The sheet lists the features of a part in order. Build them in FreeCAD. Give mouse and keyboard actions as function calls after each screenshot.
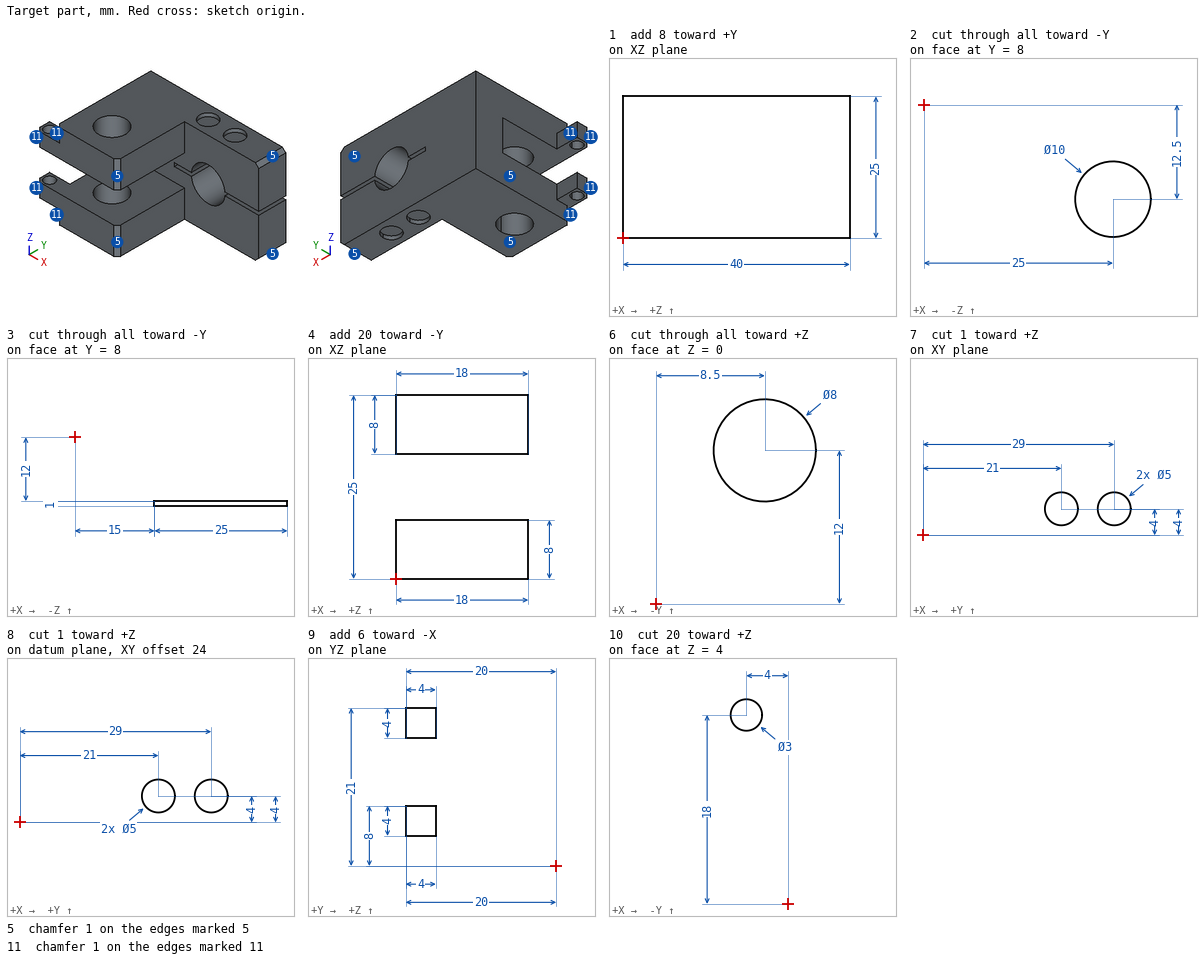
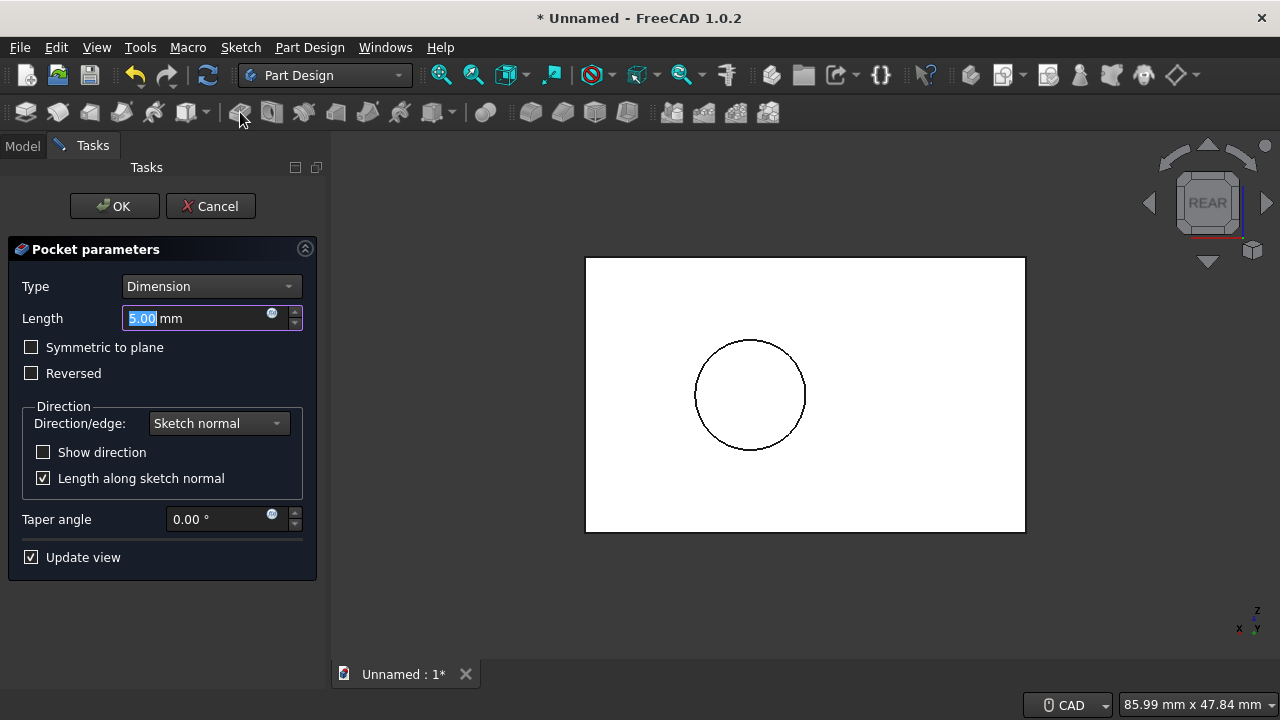
click(212, 286)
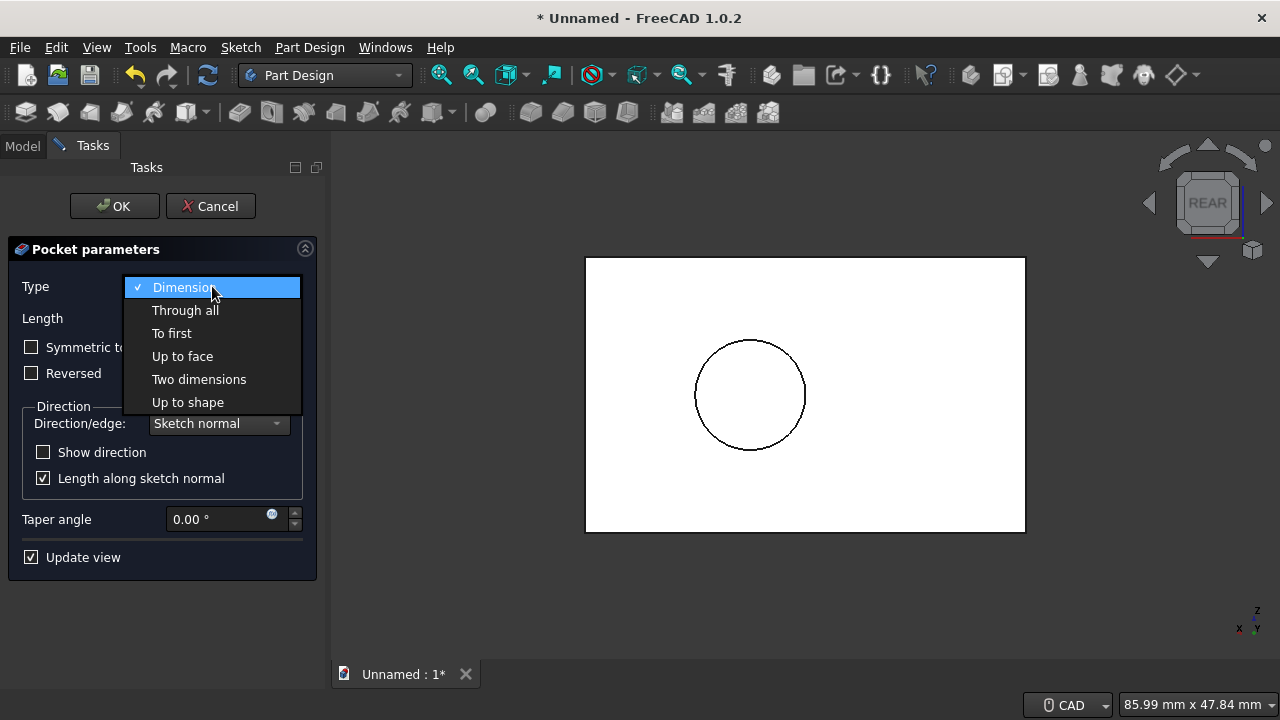
click(212, 310)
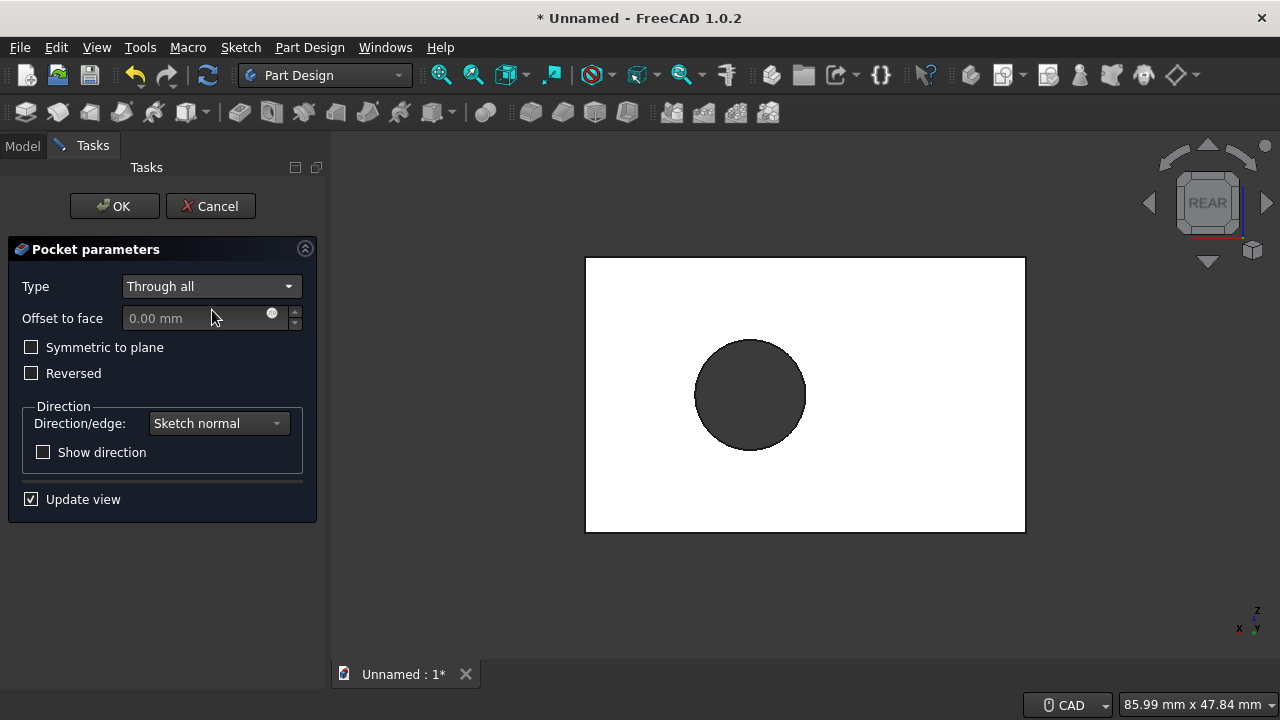
click(115, 206)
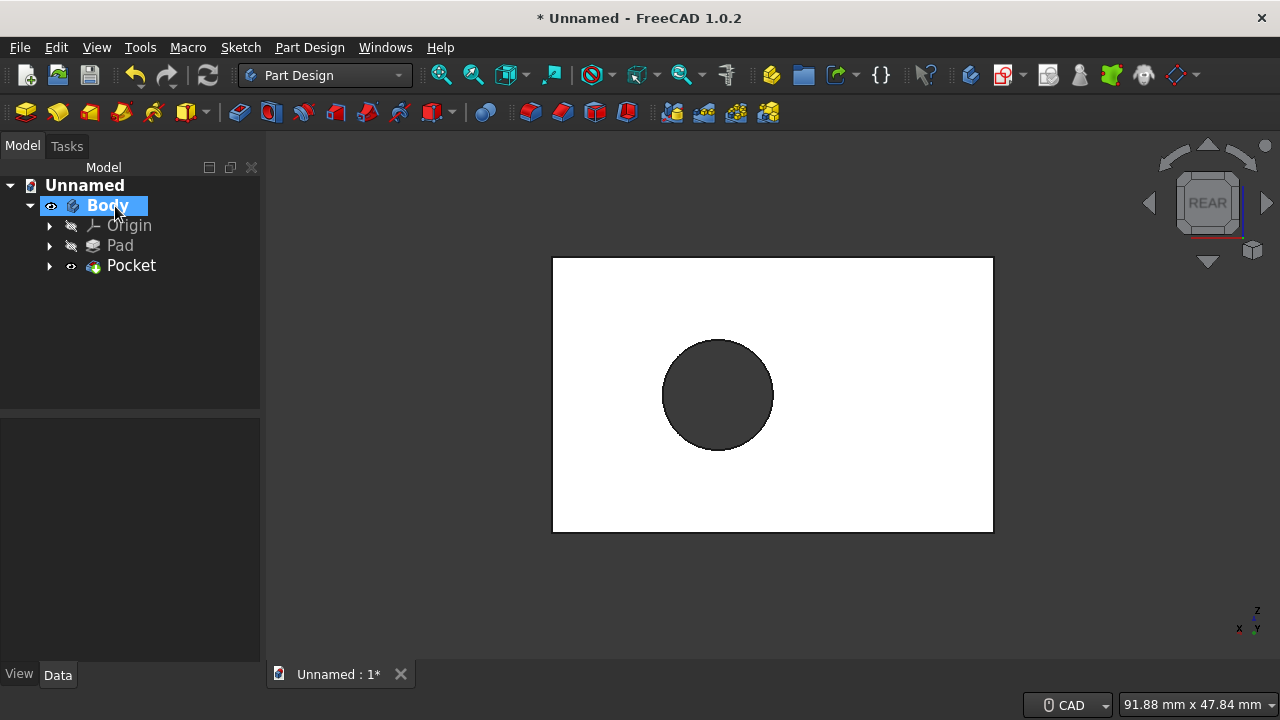
click(899, 355)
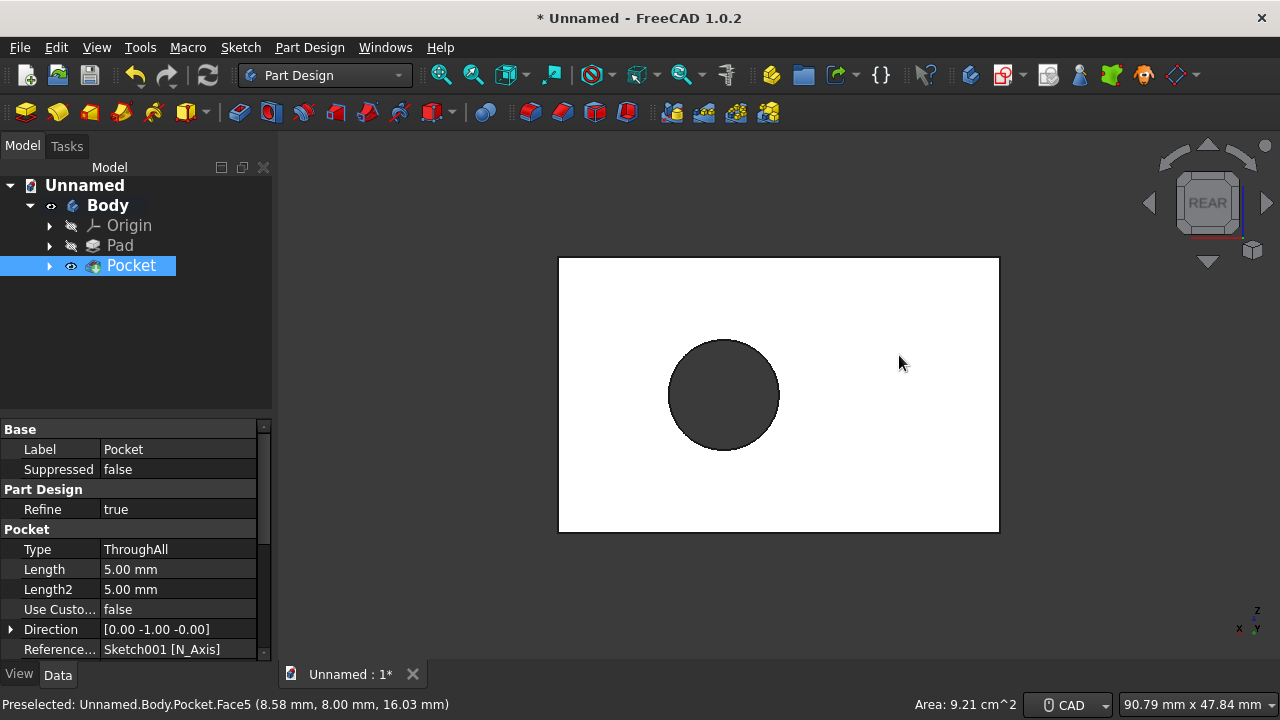
click(1004, 76)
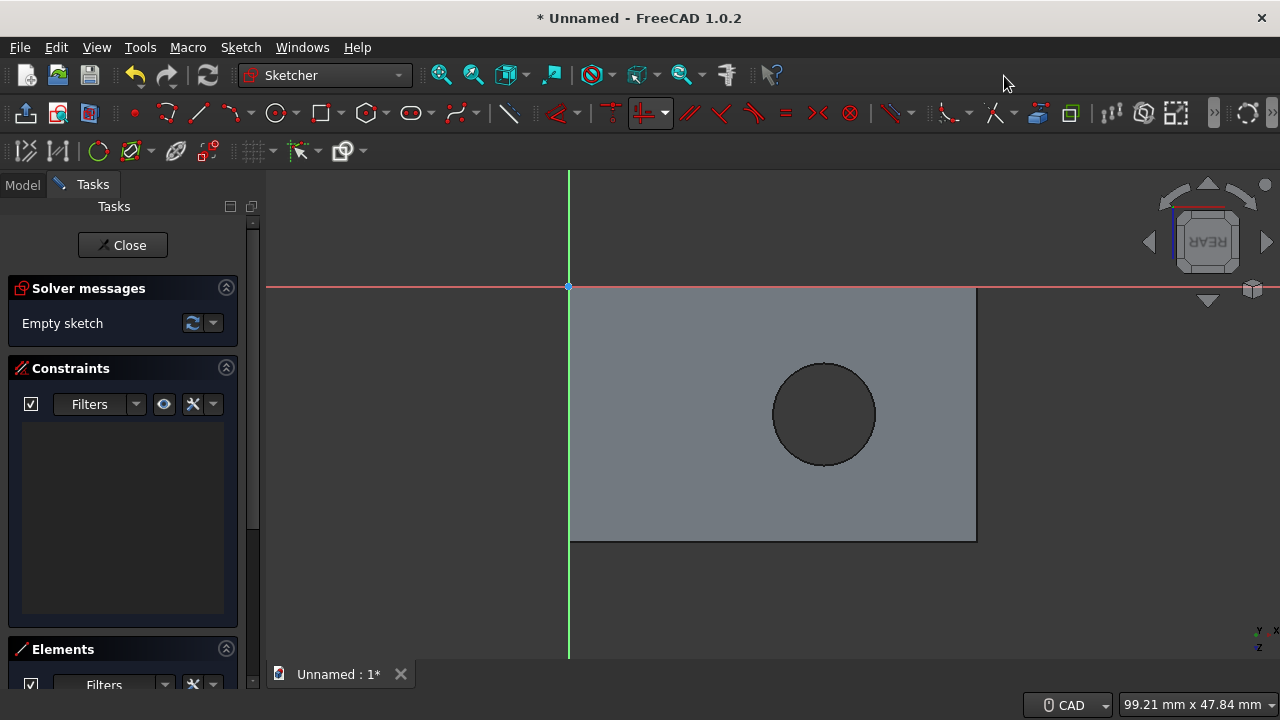
scroll(912, 228, up, 2)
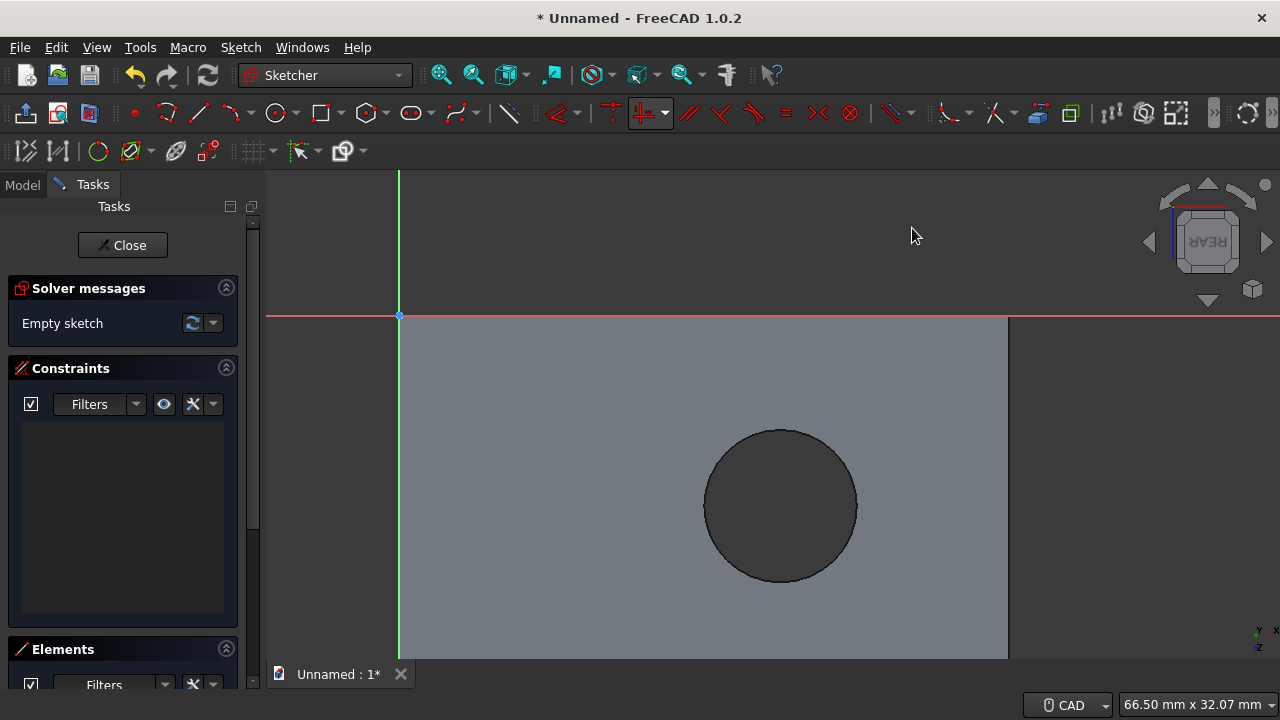
click(322, 114)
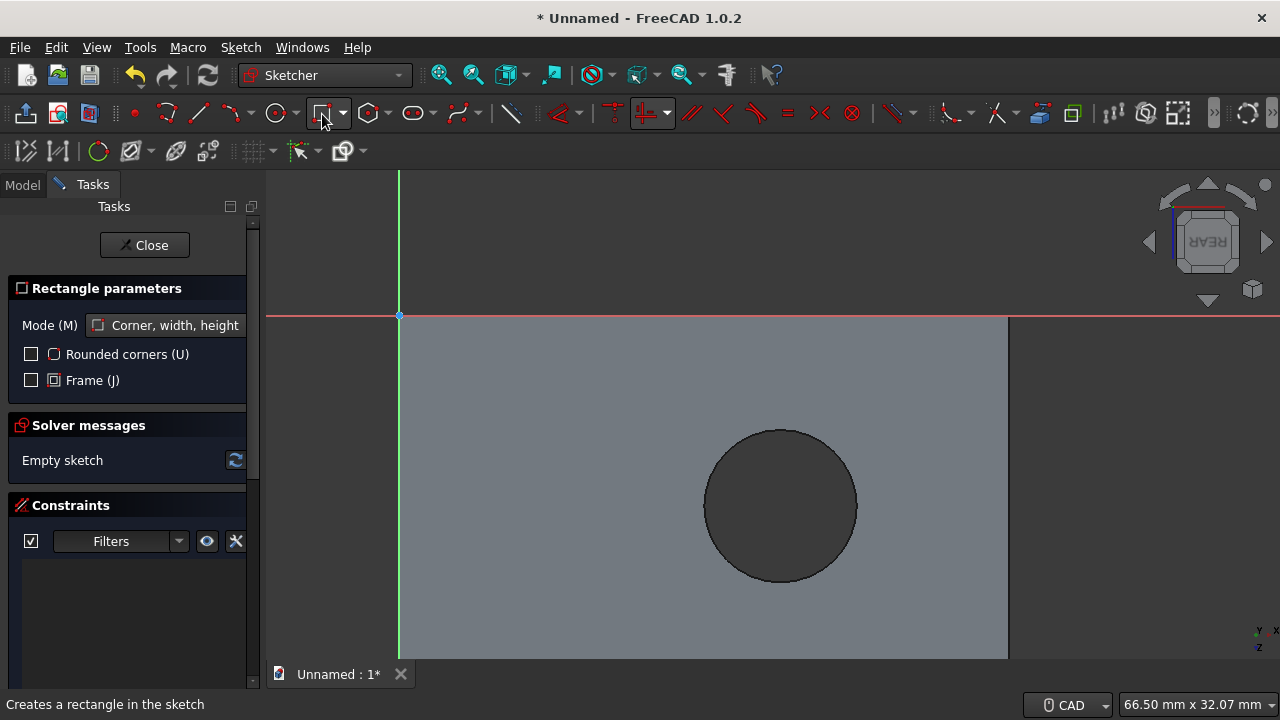
click(628, 499)
click(1009, 514)
key(Escape)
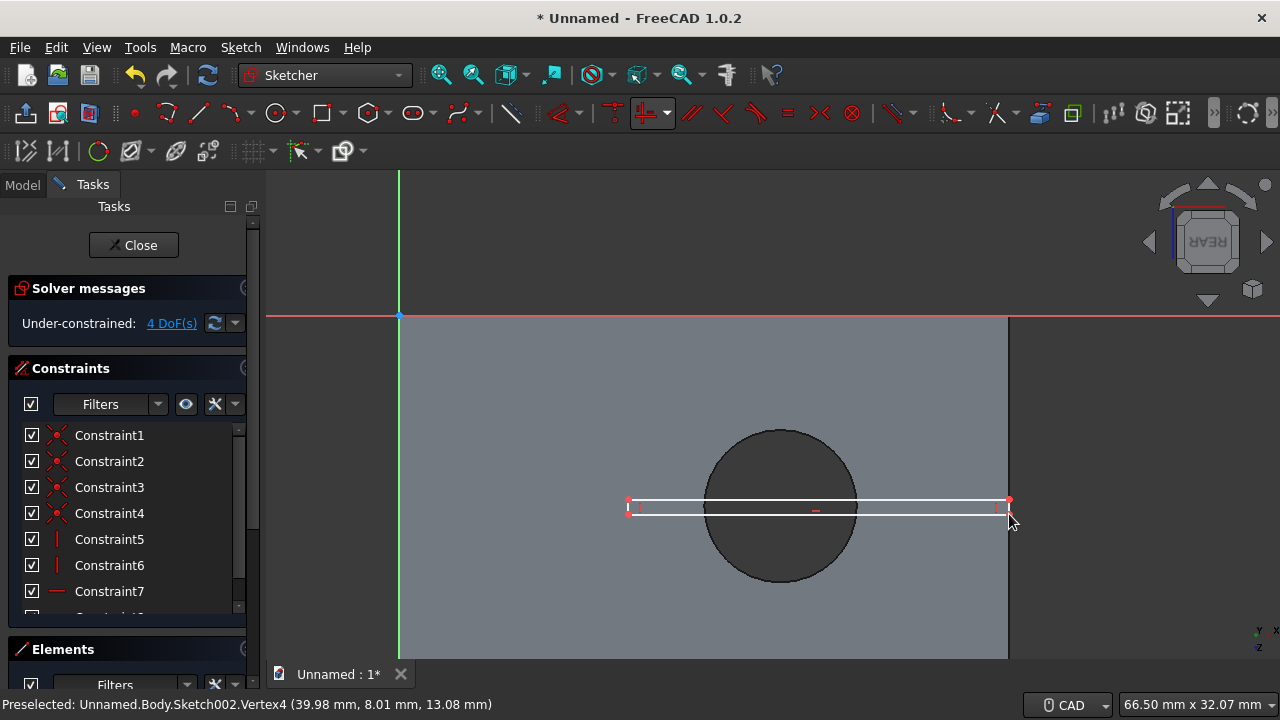
click(558, 114)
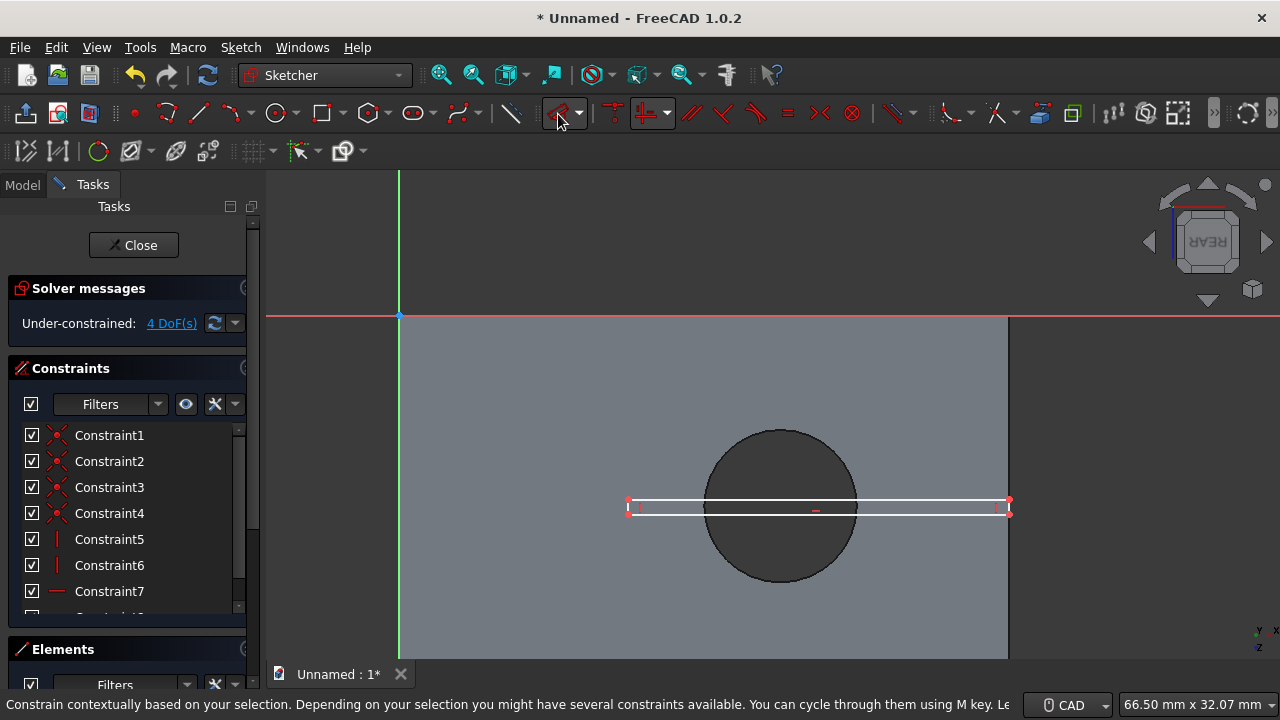
scroll(628, 508, up, 5)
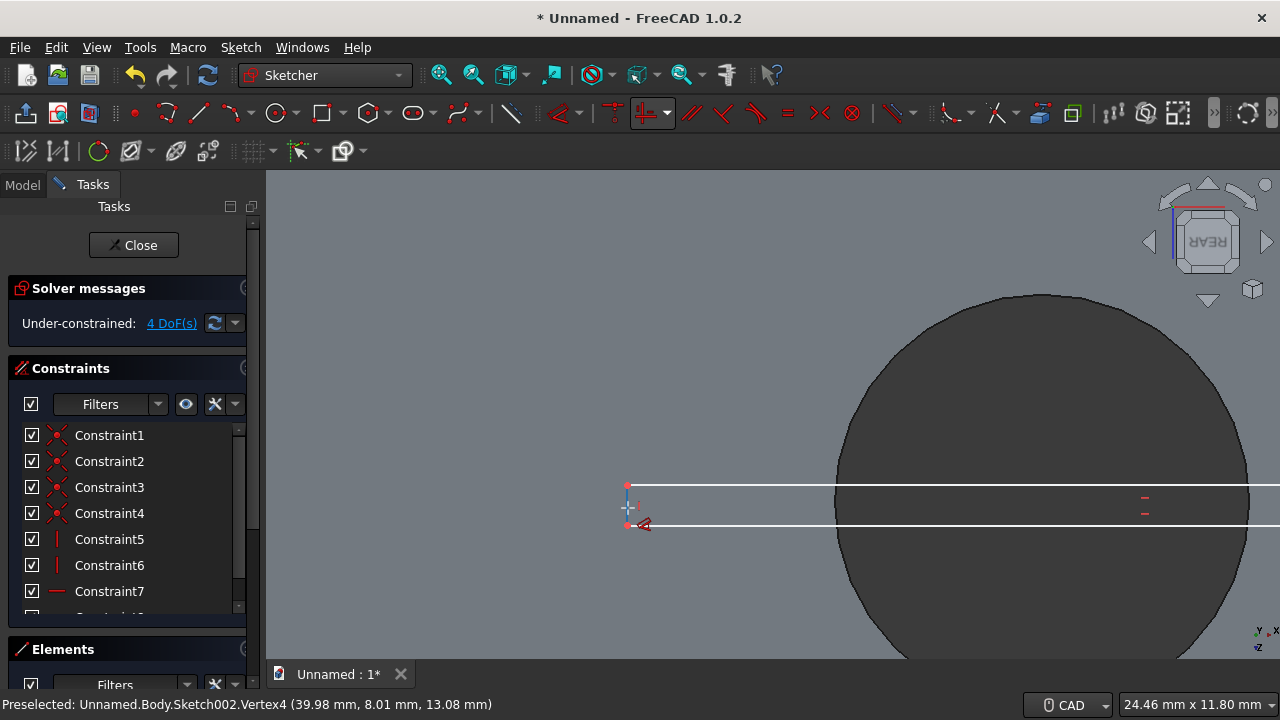
click(627, 505)
click(593, 505)